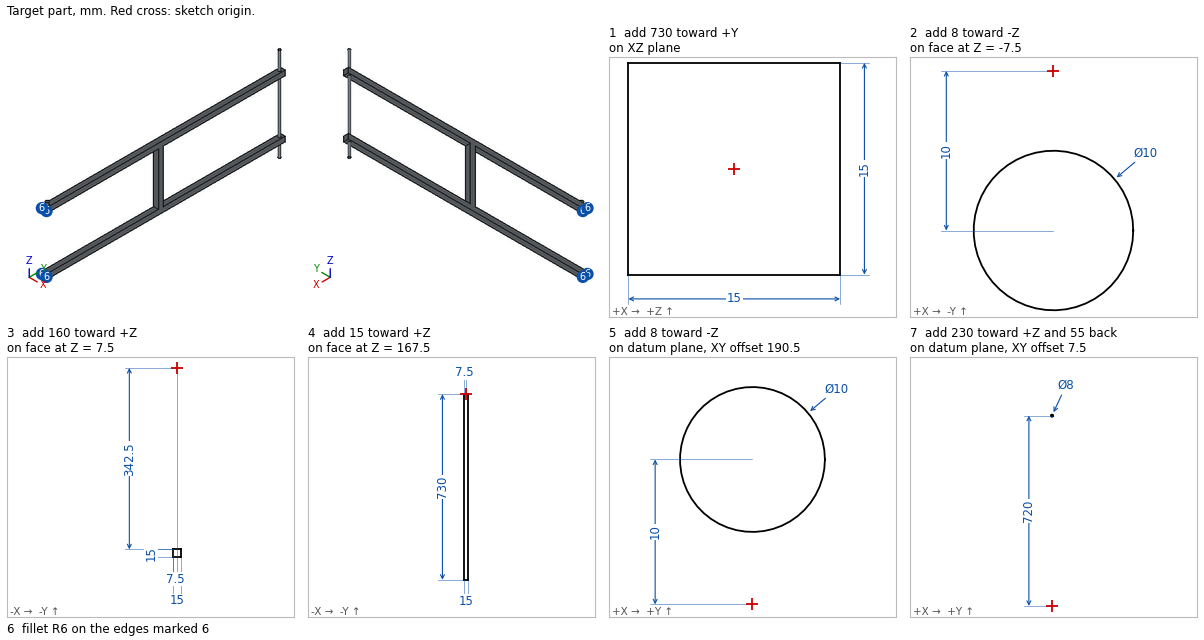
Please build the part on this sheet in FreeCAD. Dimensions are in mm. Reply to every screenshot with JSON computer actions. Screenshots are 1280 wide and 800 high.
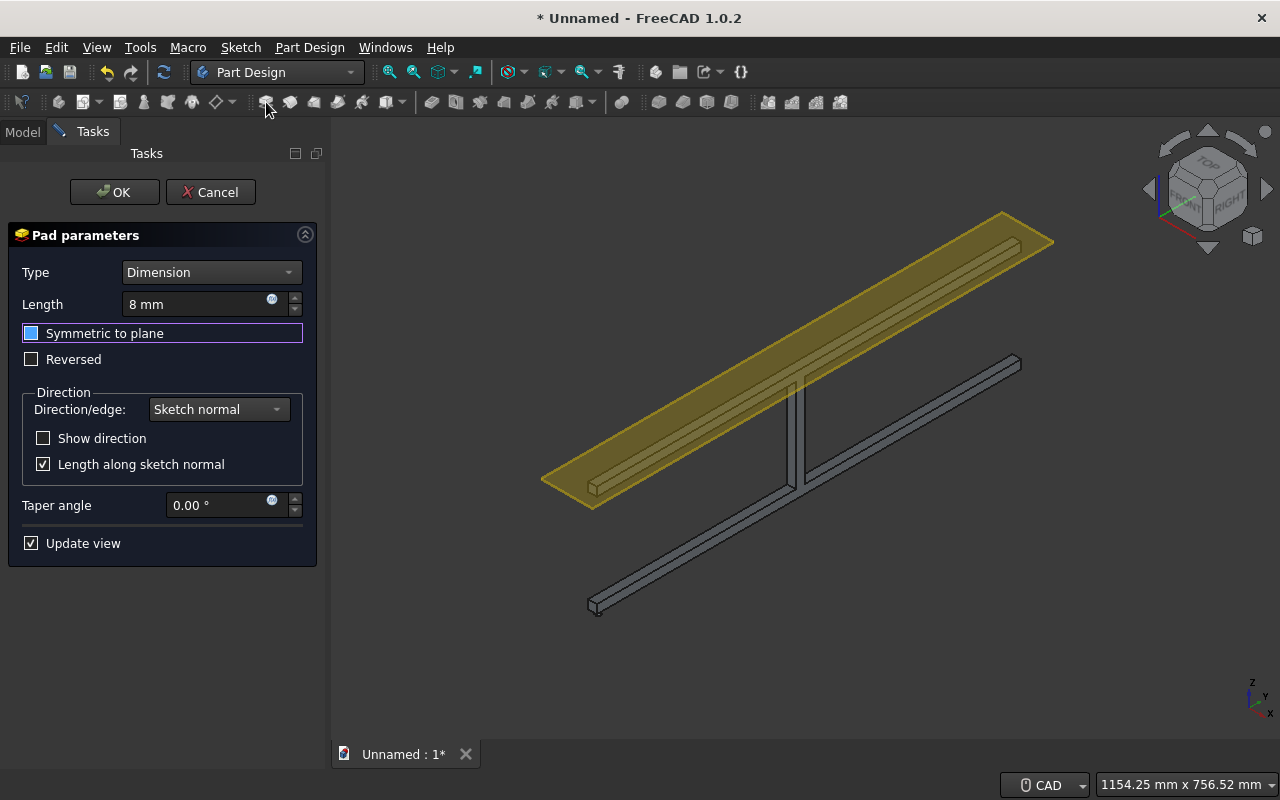
{"action": "left_click", "coordinate": [30, 359]}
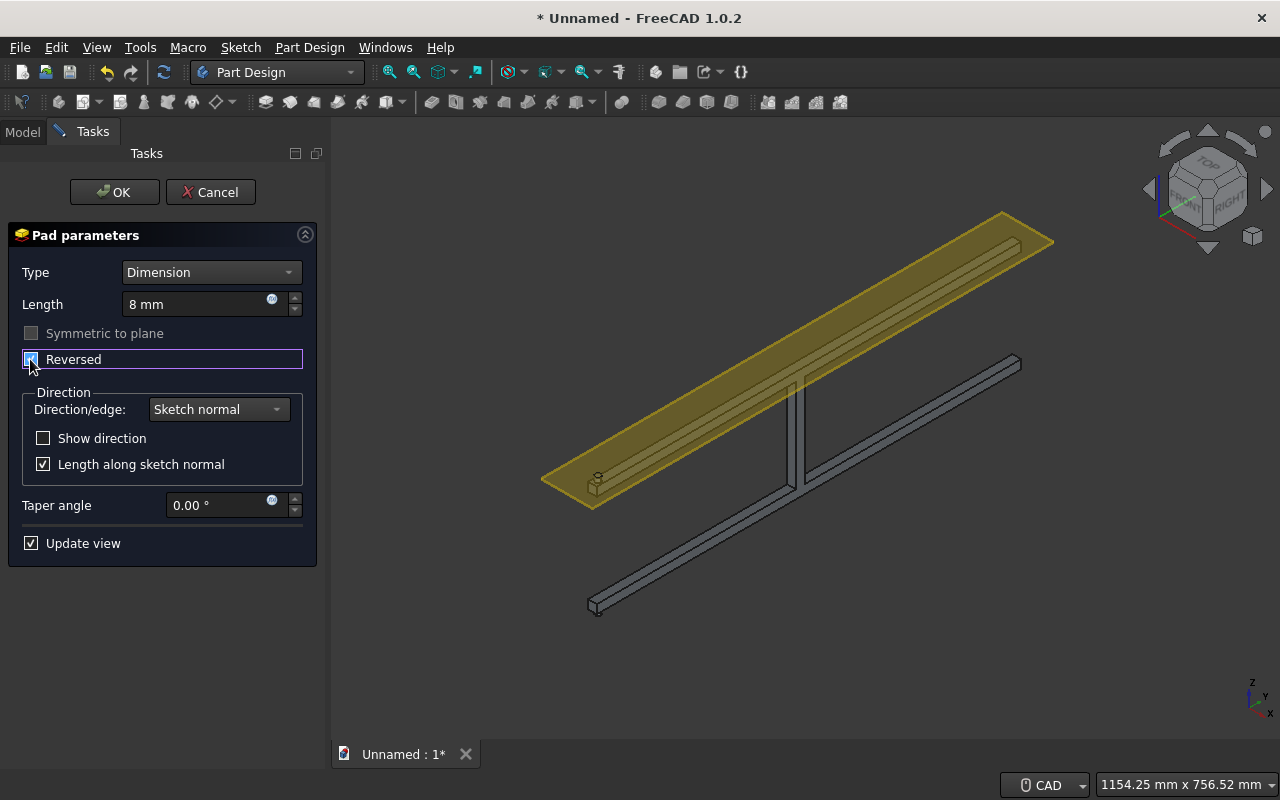
{"action": "left_click", "coordinate": [115, 192]}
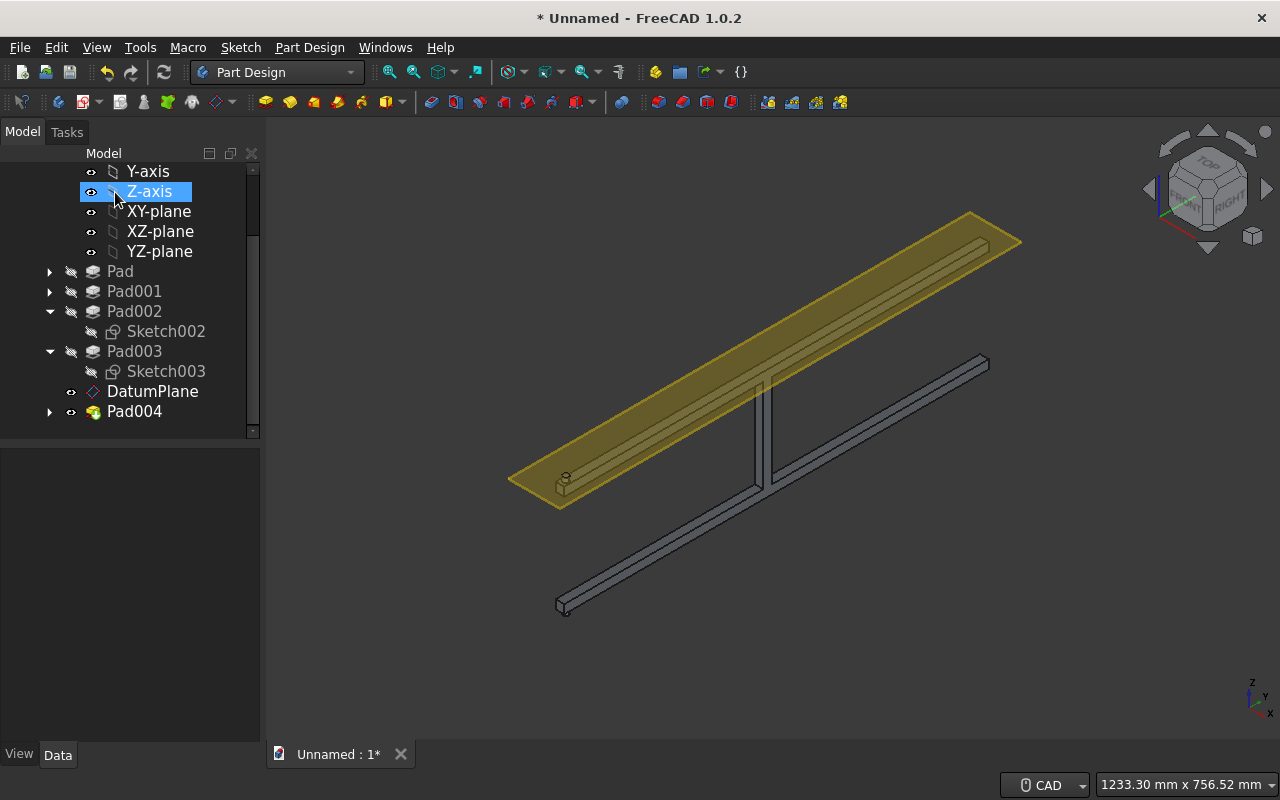
{"action": "left_click", "coordinate": [116, 392]}
{"action": "key", "text": "space"}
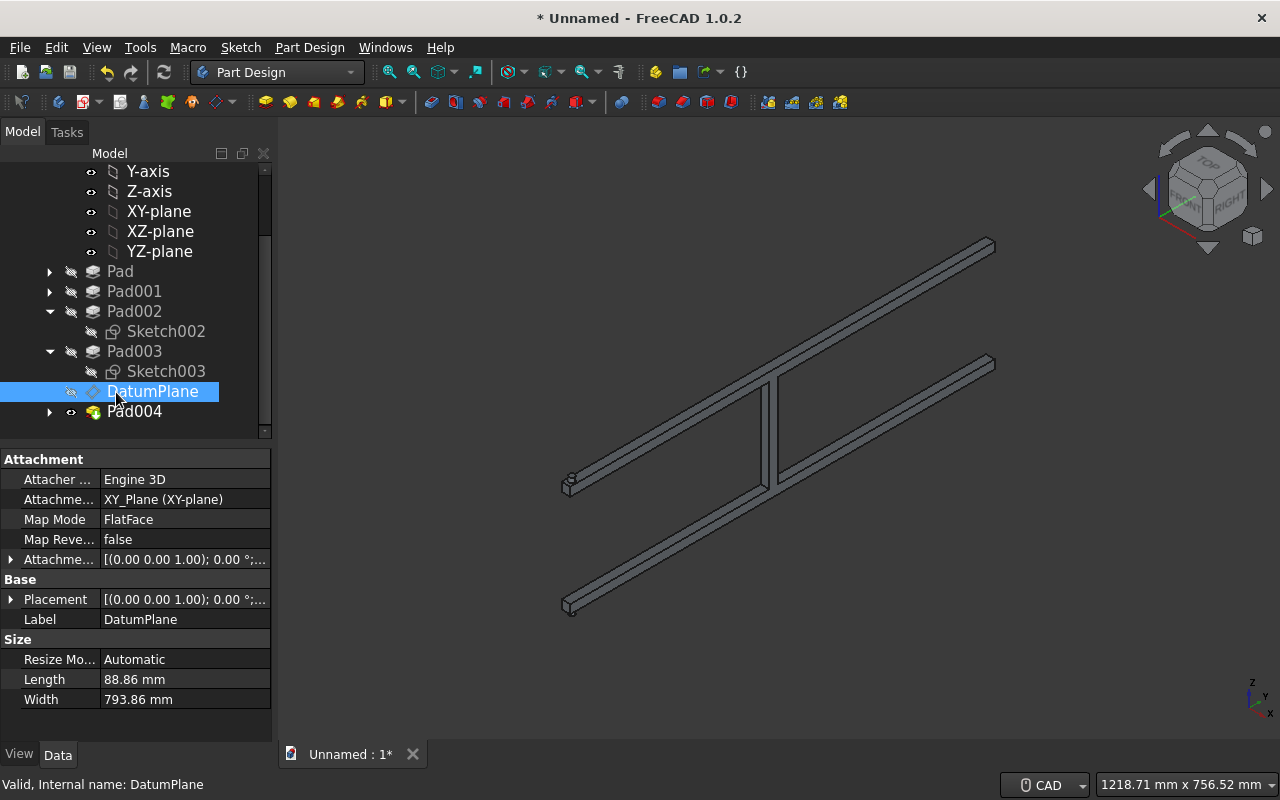
{"action": "left_click", "coordinate": [570, 492]}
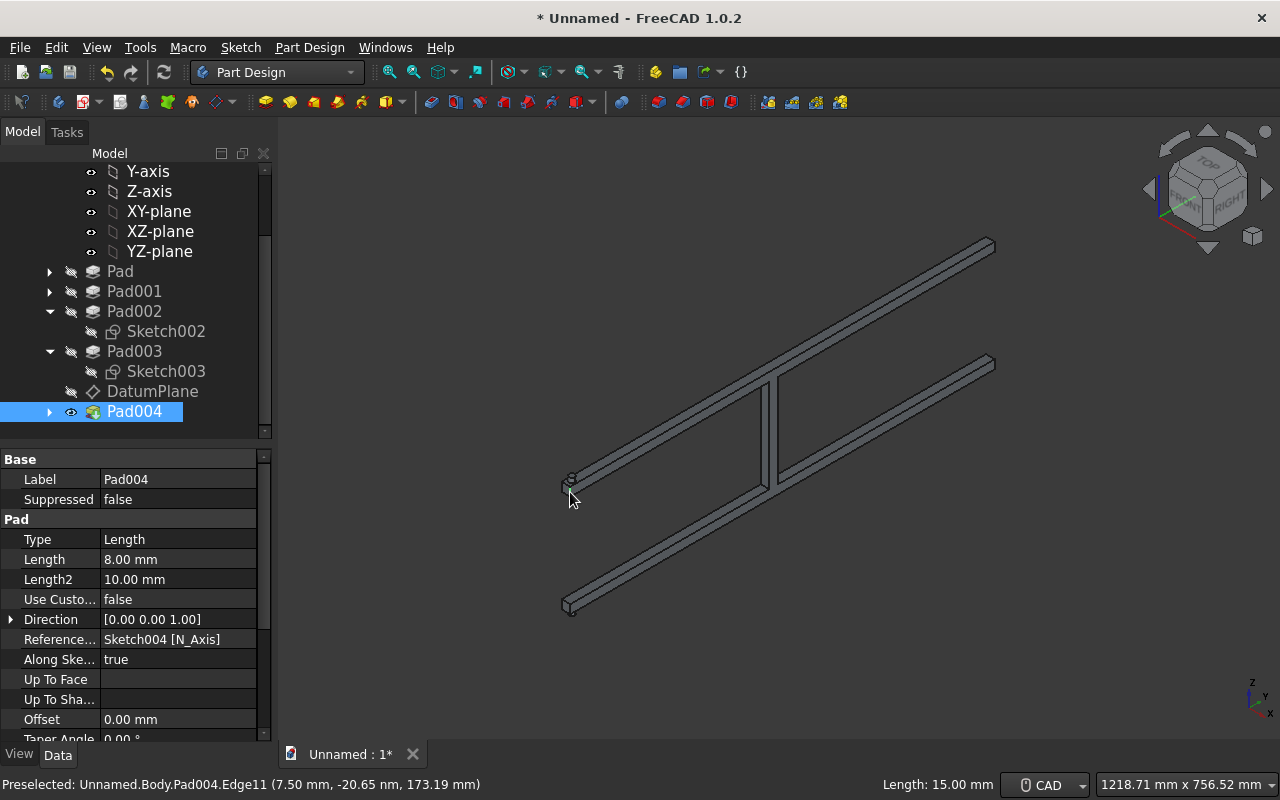
{"action": "left_click", "coordinate": [570, 610], "text": "ctrl"}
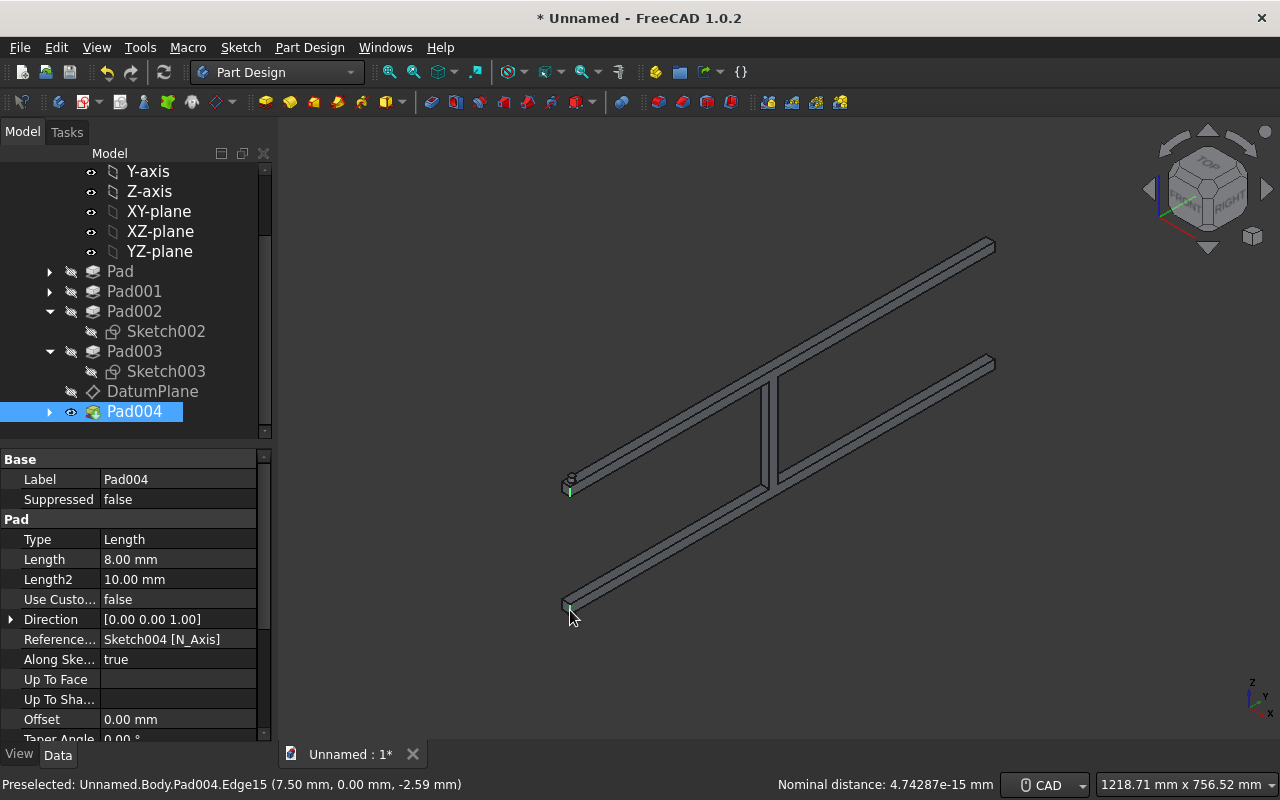
{"action": "scroll", "coordinate": [562, 486], "scroll_direction": "up", "scroll_amount": 6}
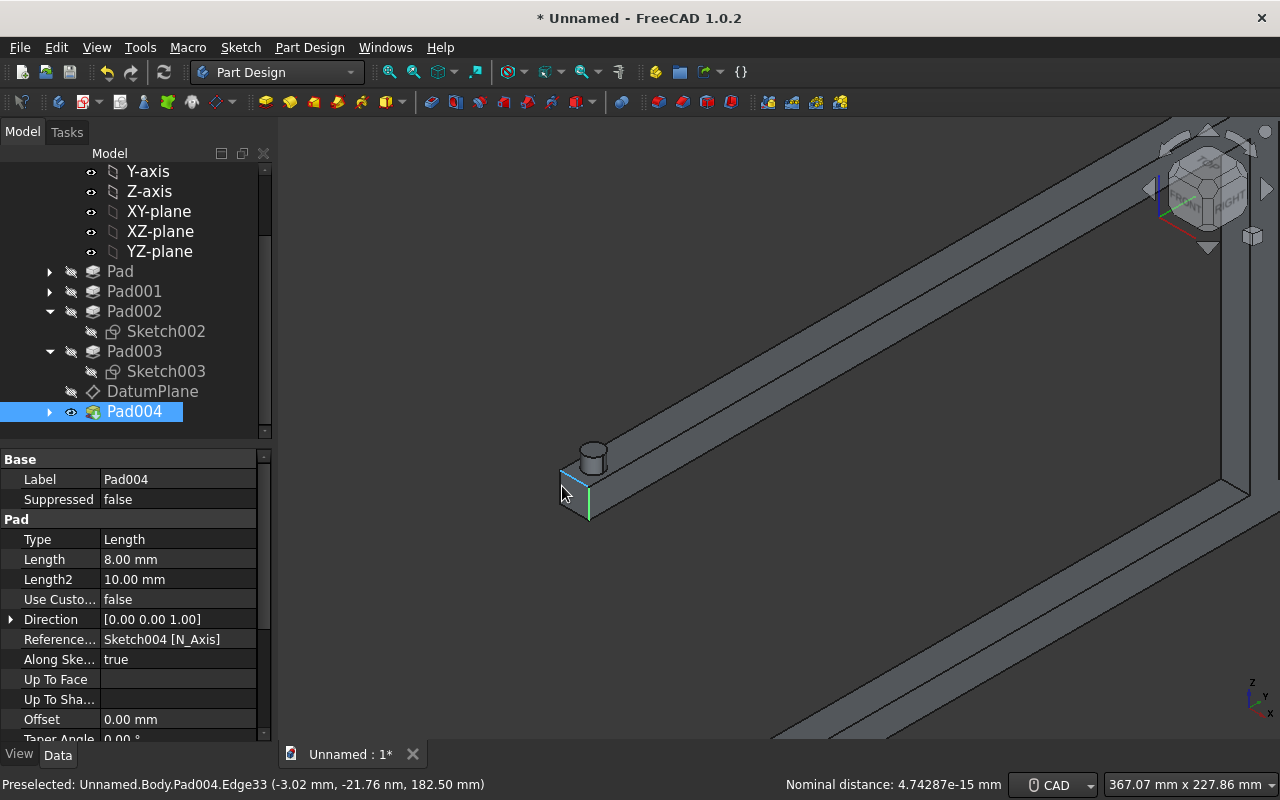
{"action": "left_click", "coordinate": [390, 72]}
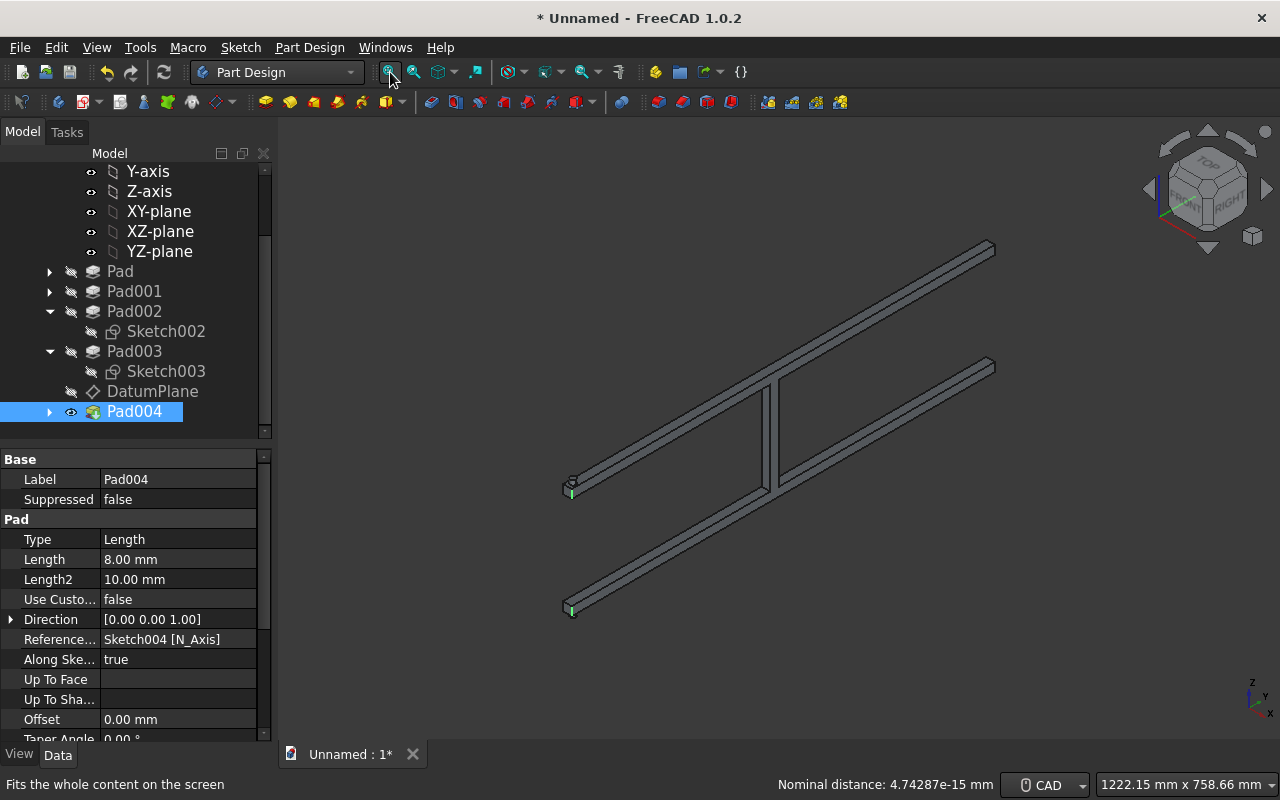
{"action": "key", "text": "2"}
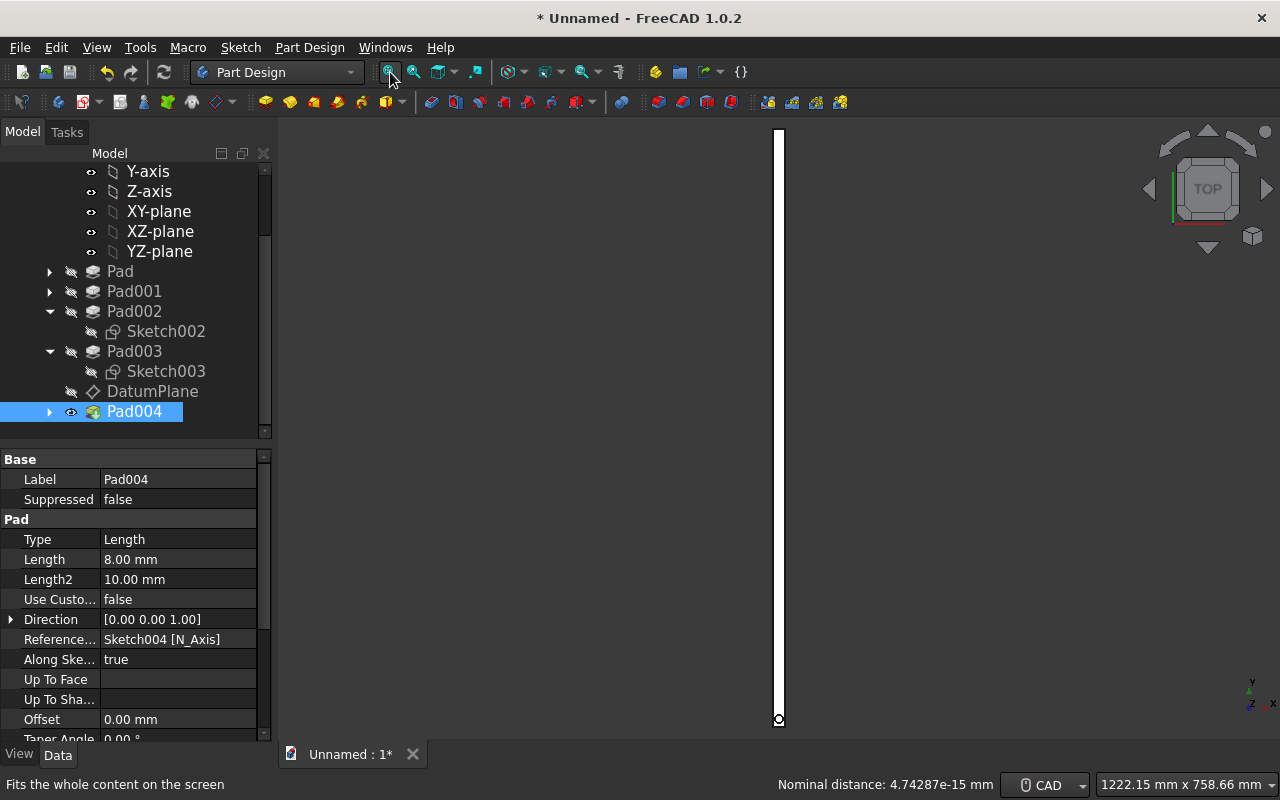
{"action": "key", "text": "0"}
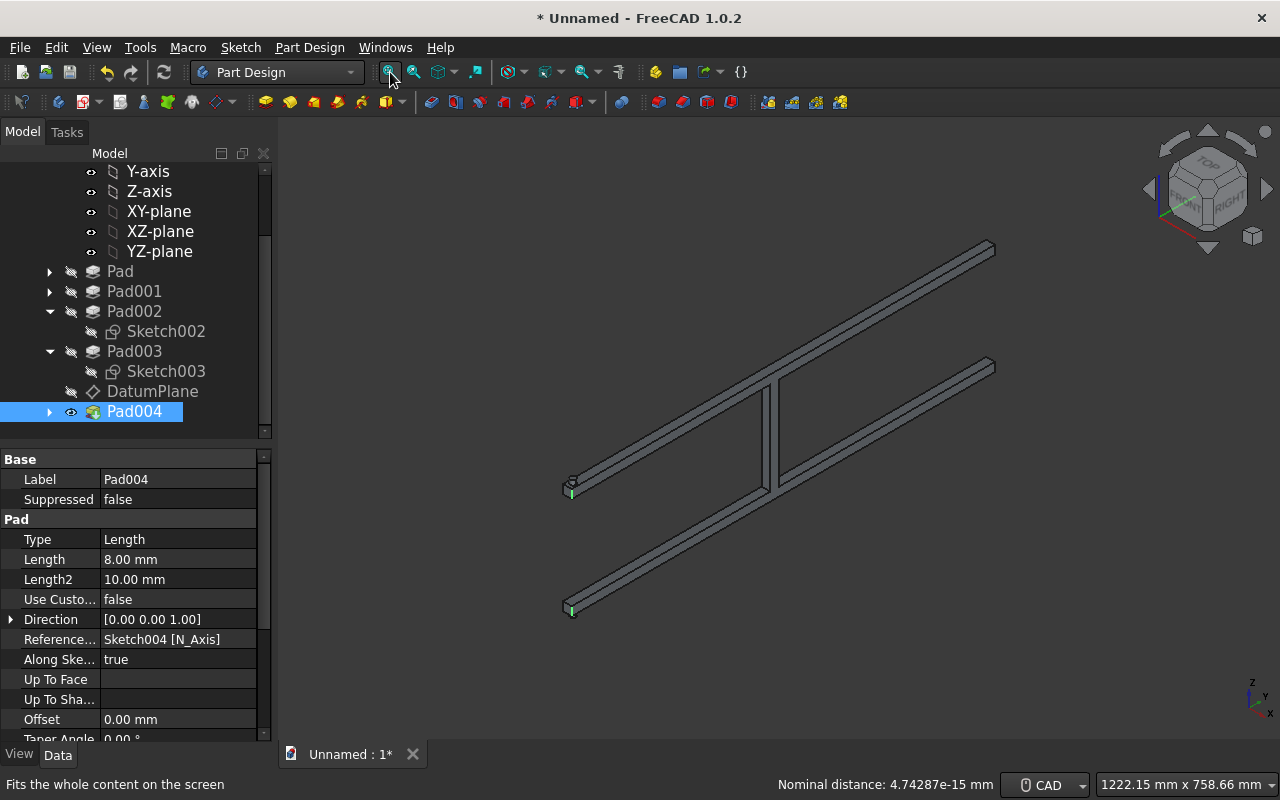
{"action": "scroll", "coordinate": [563, 488], "scroll_direction": "up", "scroll_amount": 6}